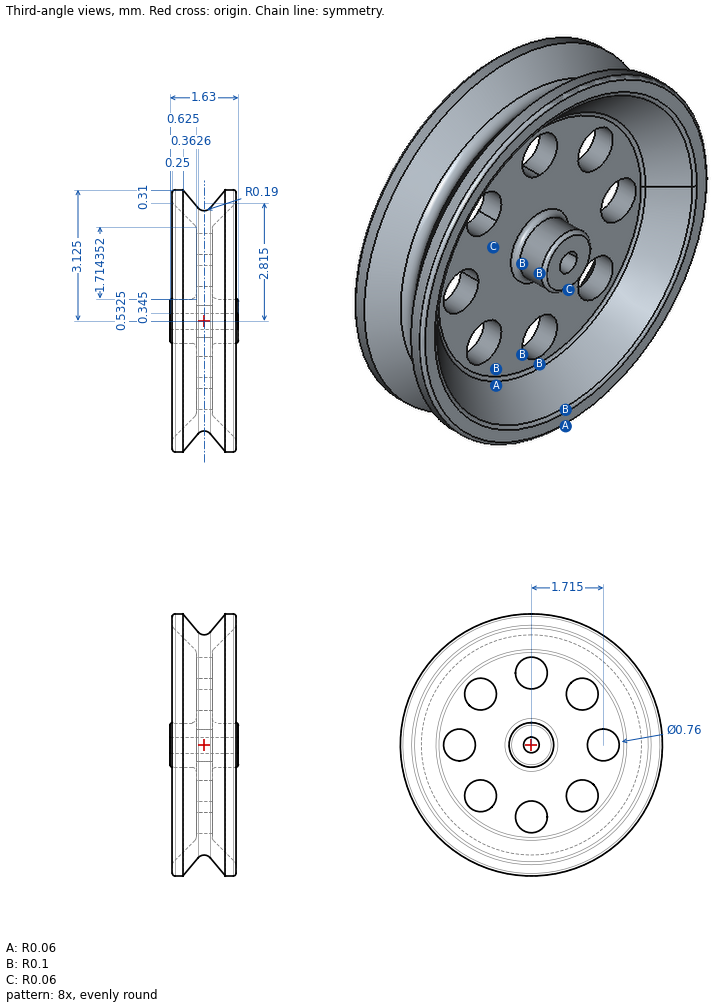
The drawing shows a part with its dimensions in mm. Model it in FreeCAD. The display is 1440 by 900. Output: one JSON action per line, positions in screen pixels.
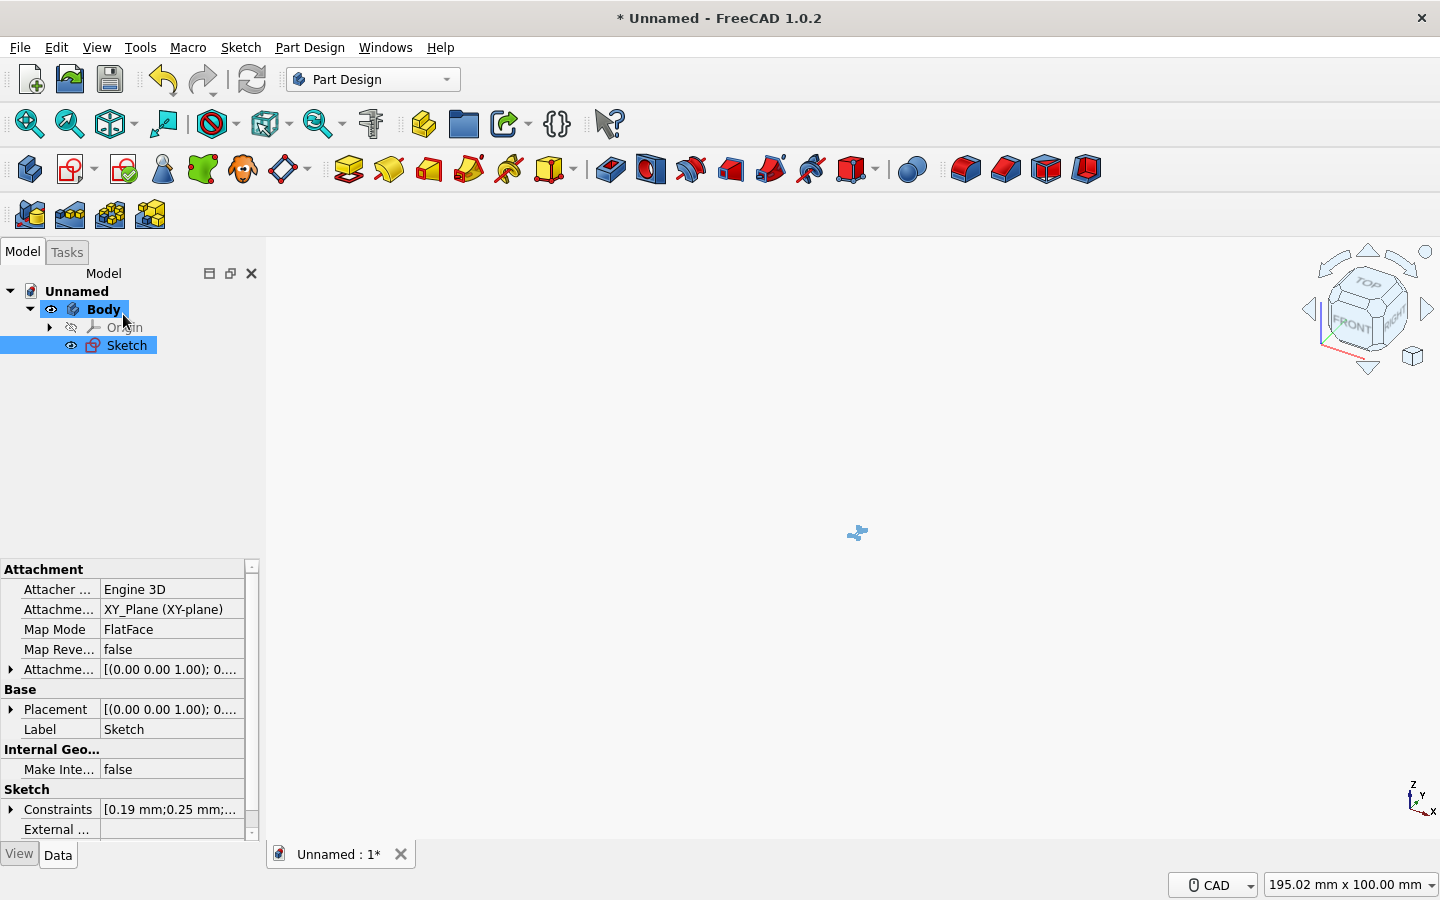
{"action": "left_click", "coordinate": [390, 170]}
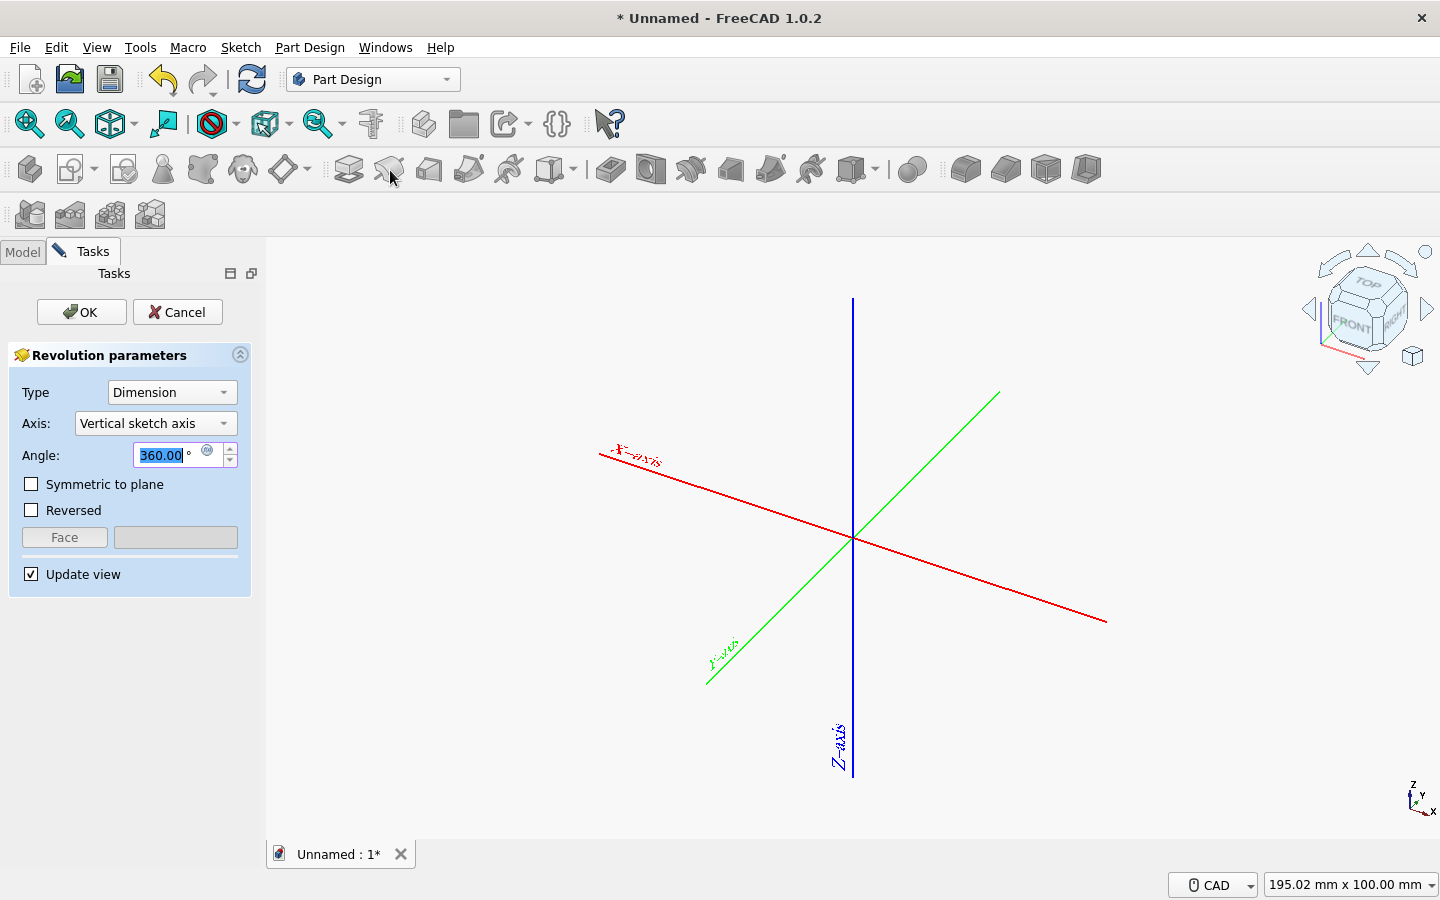
{"action": "left_click", "coordinate": [156, 424]}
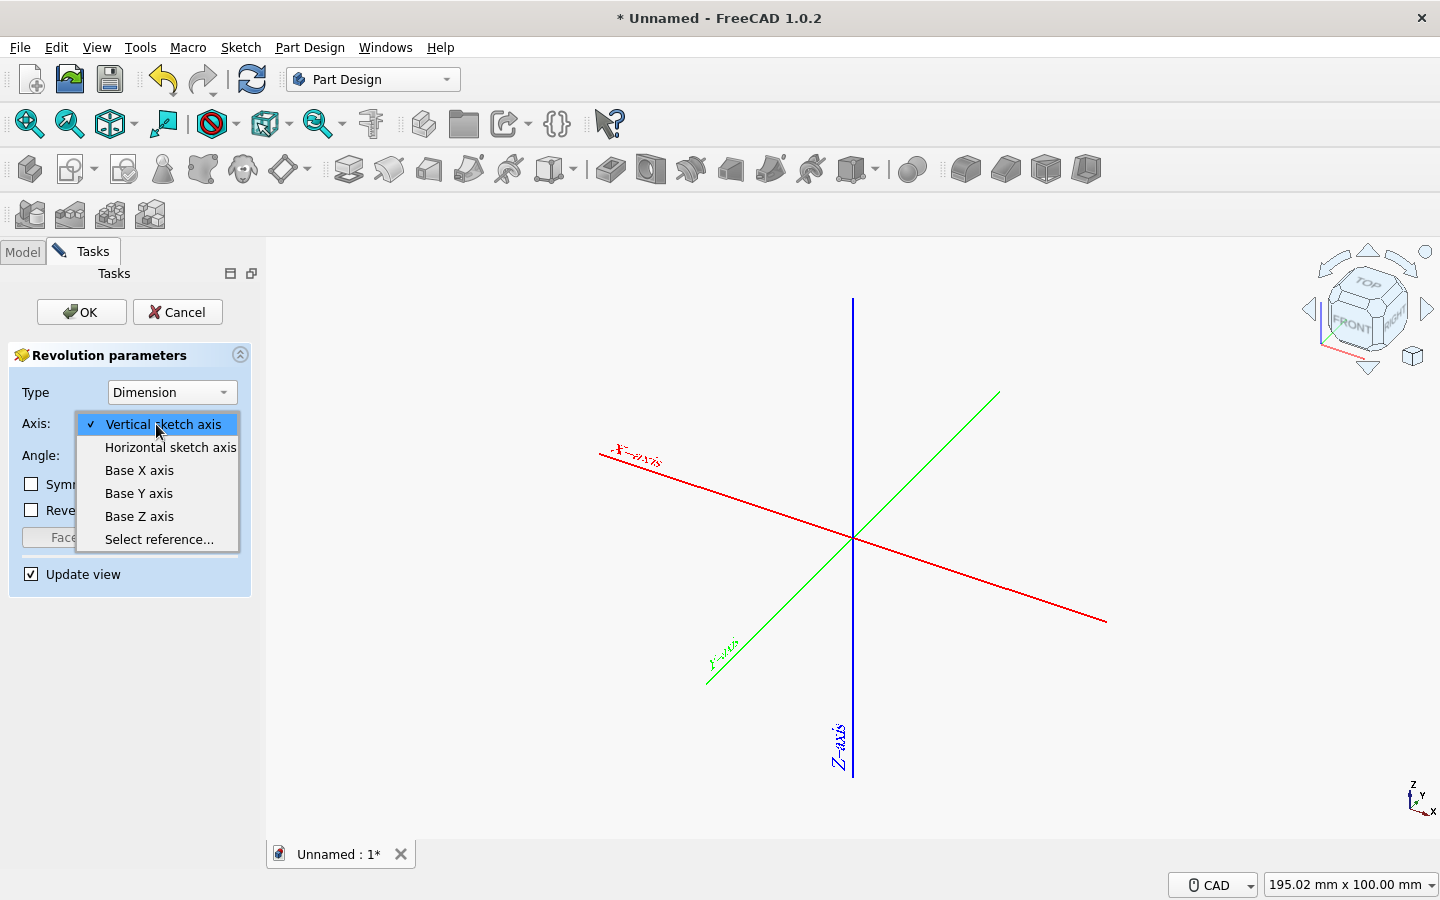
{"action": "left_click", "coordinate": [156, 448]}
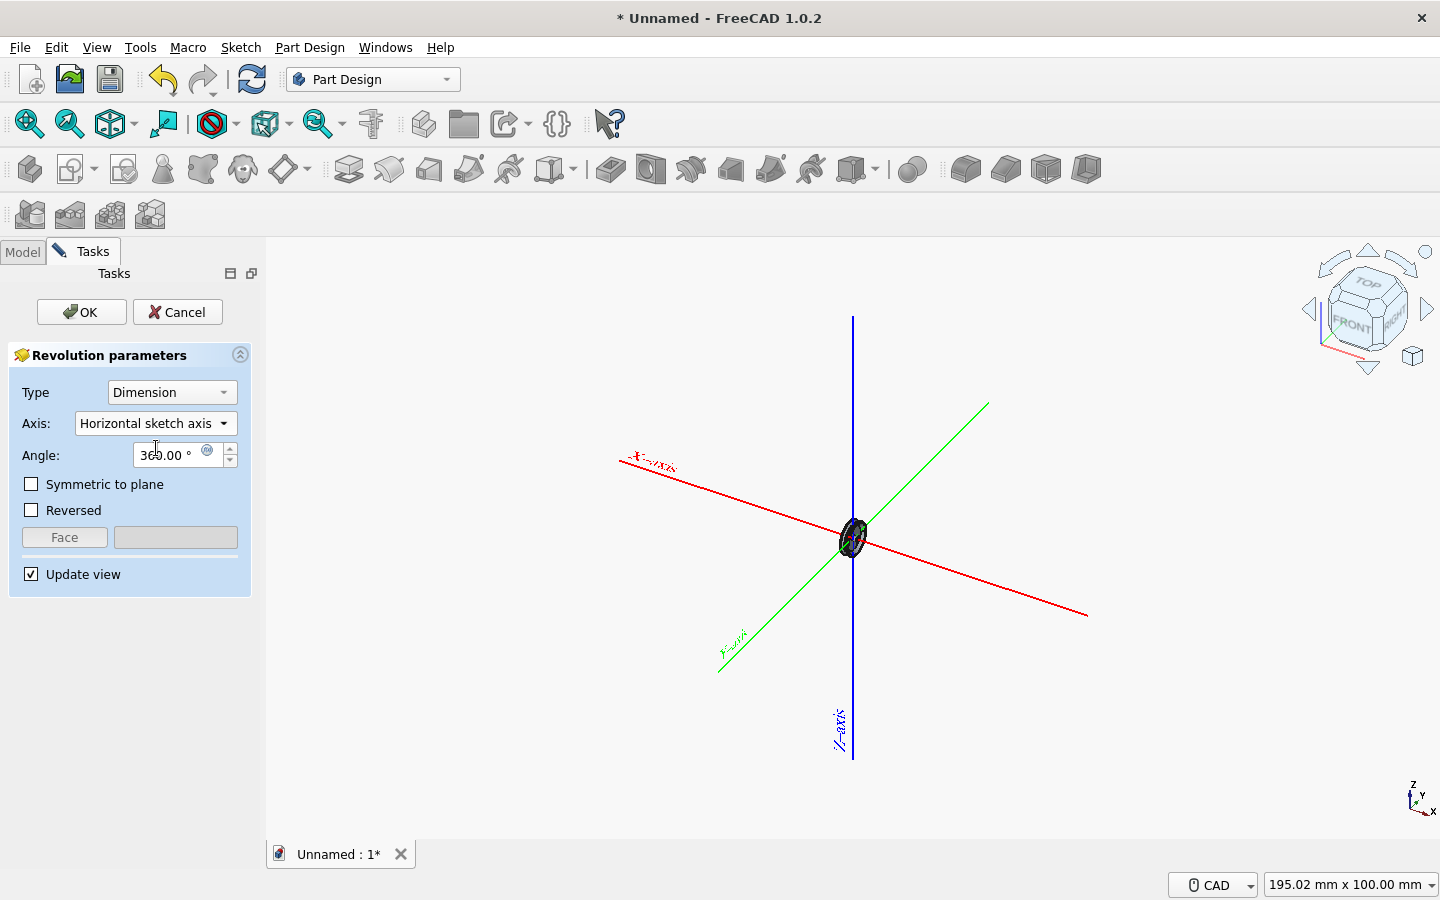
{"action": "left_click", "coordinate": [82, 312]}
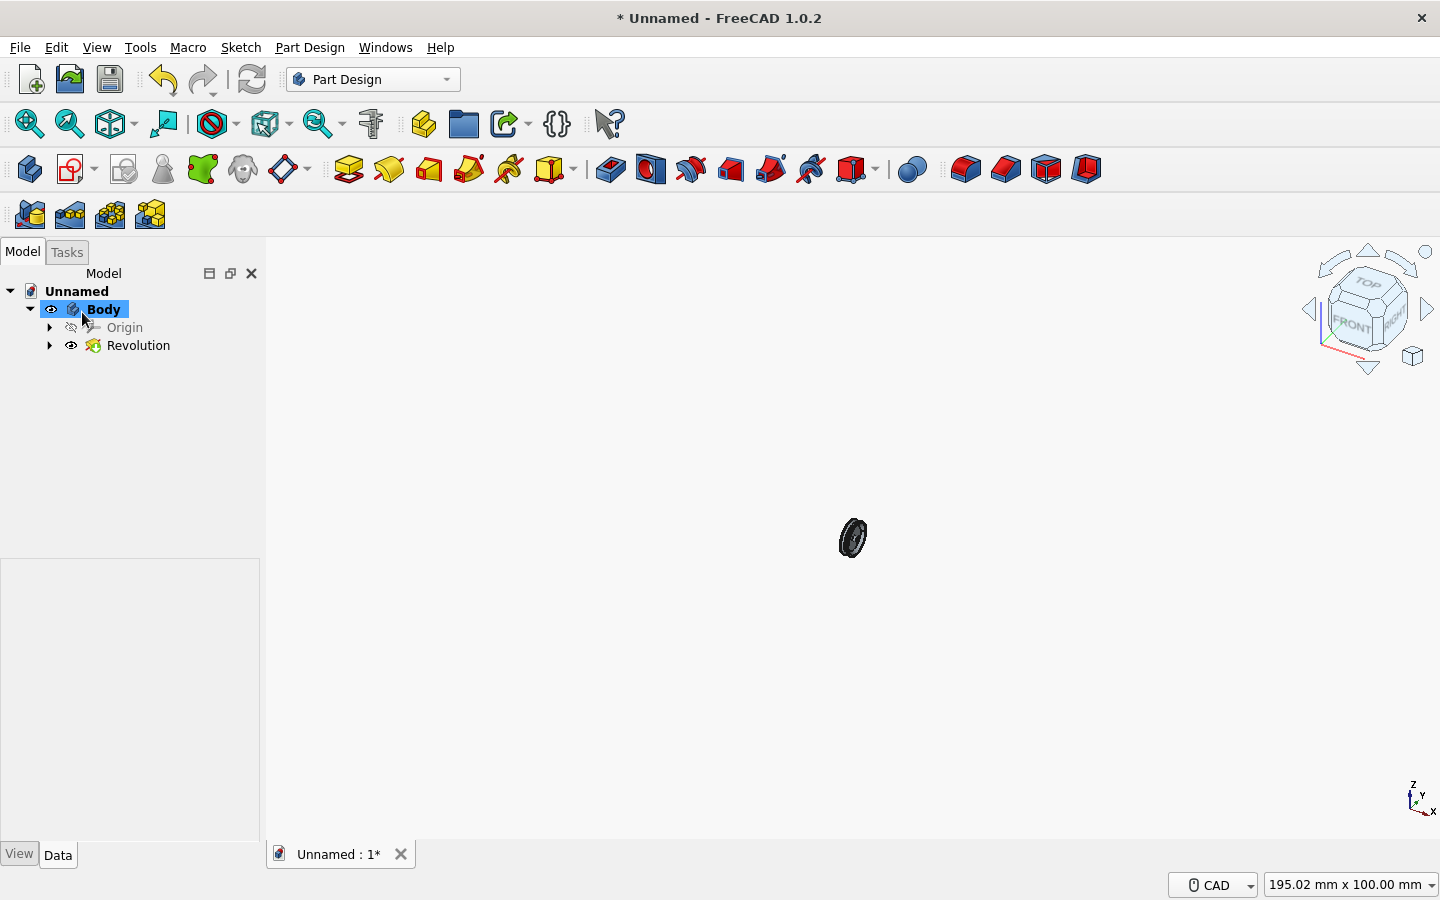
{"action": "left_click", "coordinate": [30, 124]}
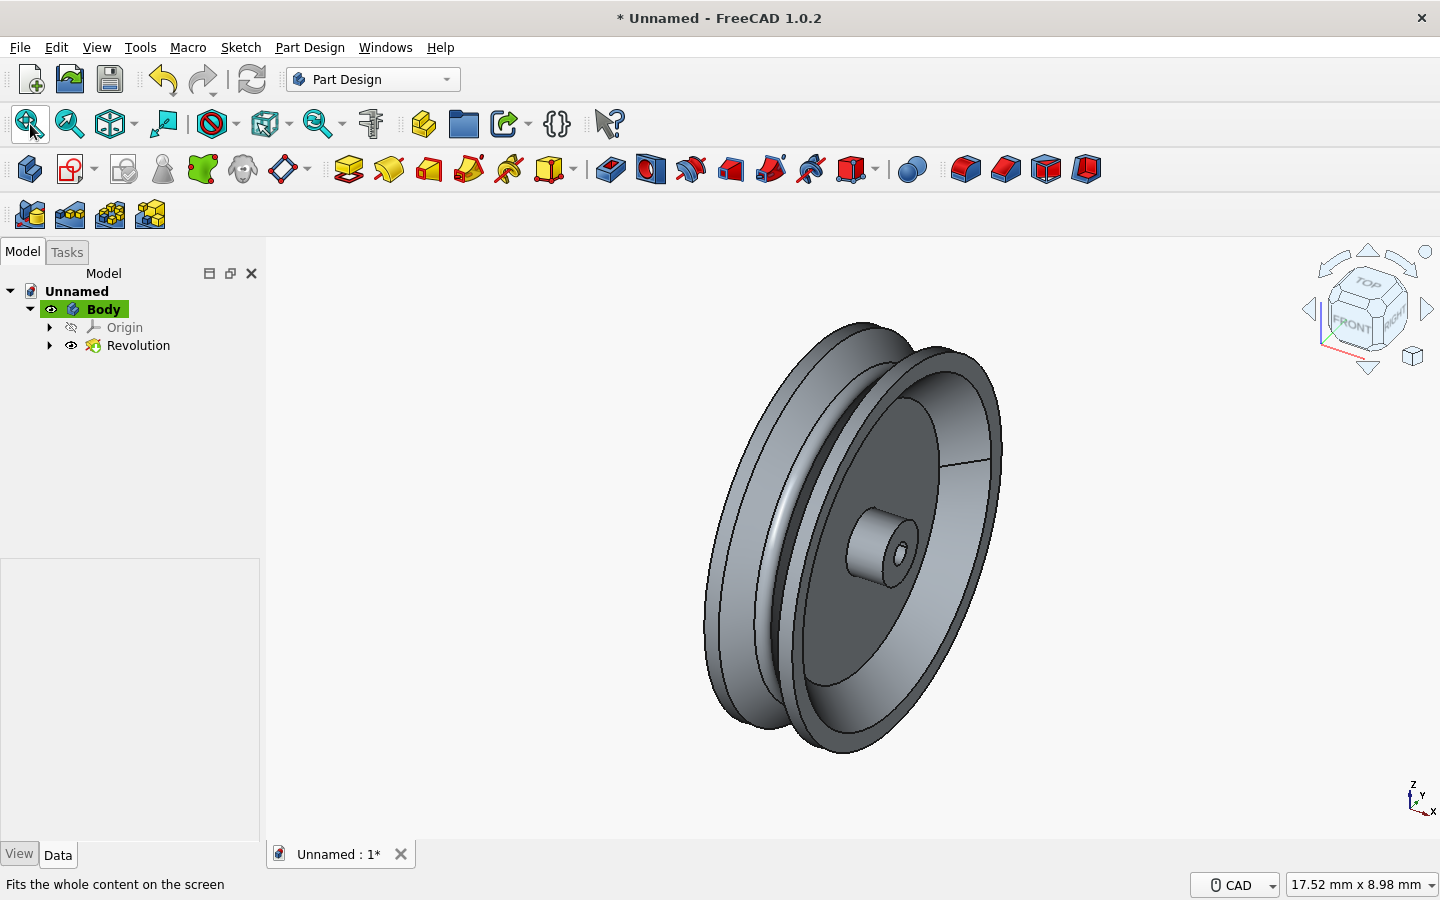
{"action": "left_click", "coordinate": [792, 656]}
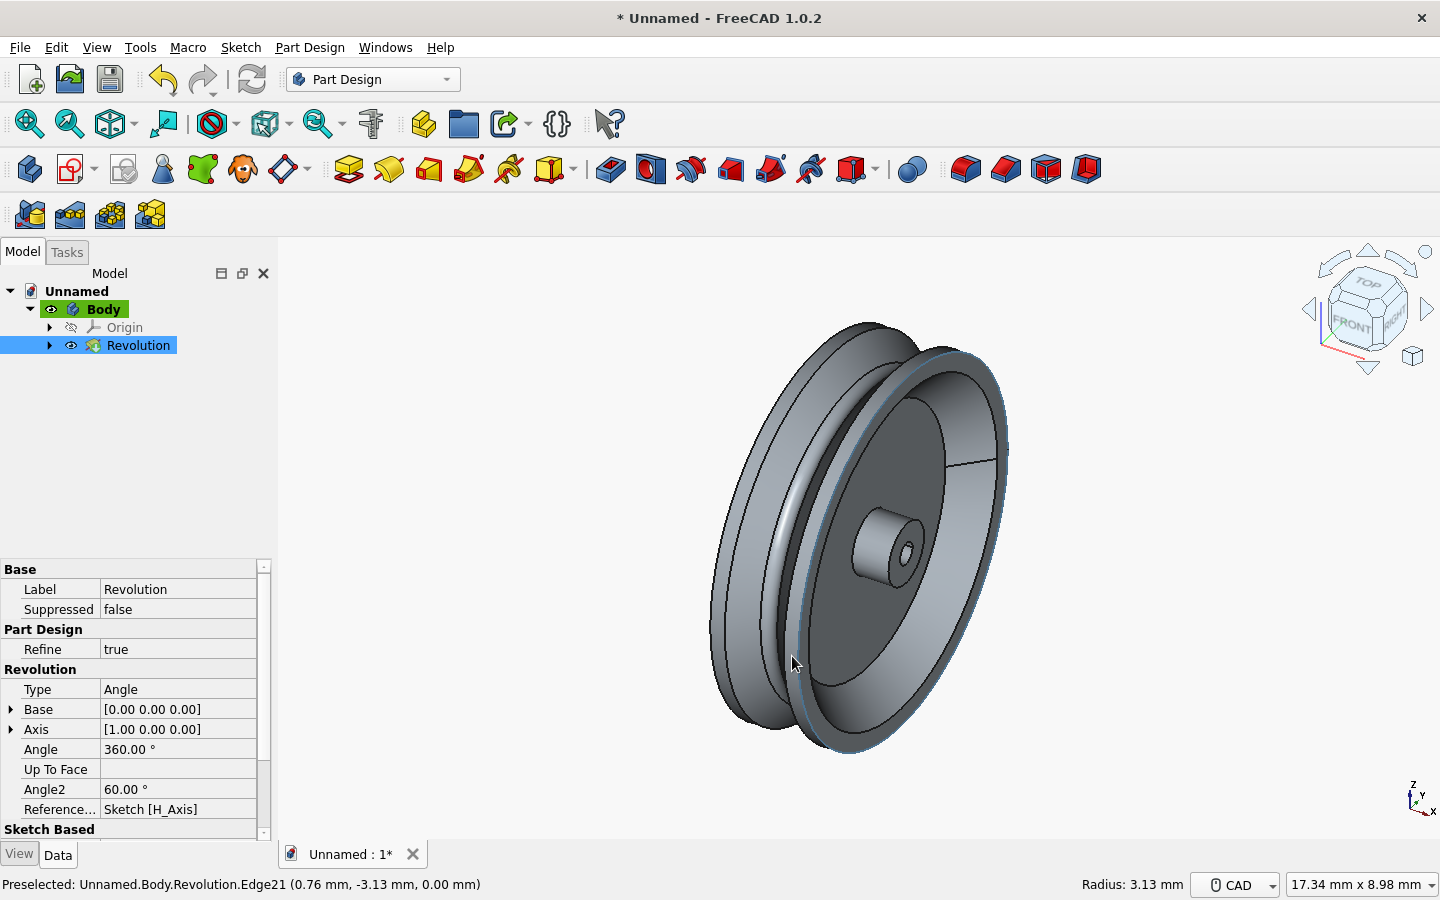
{"action": "key", "text": "0"}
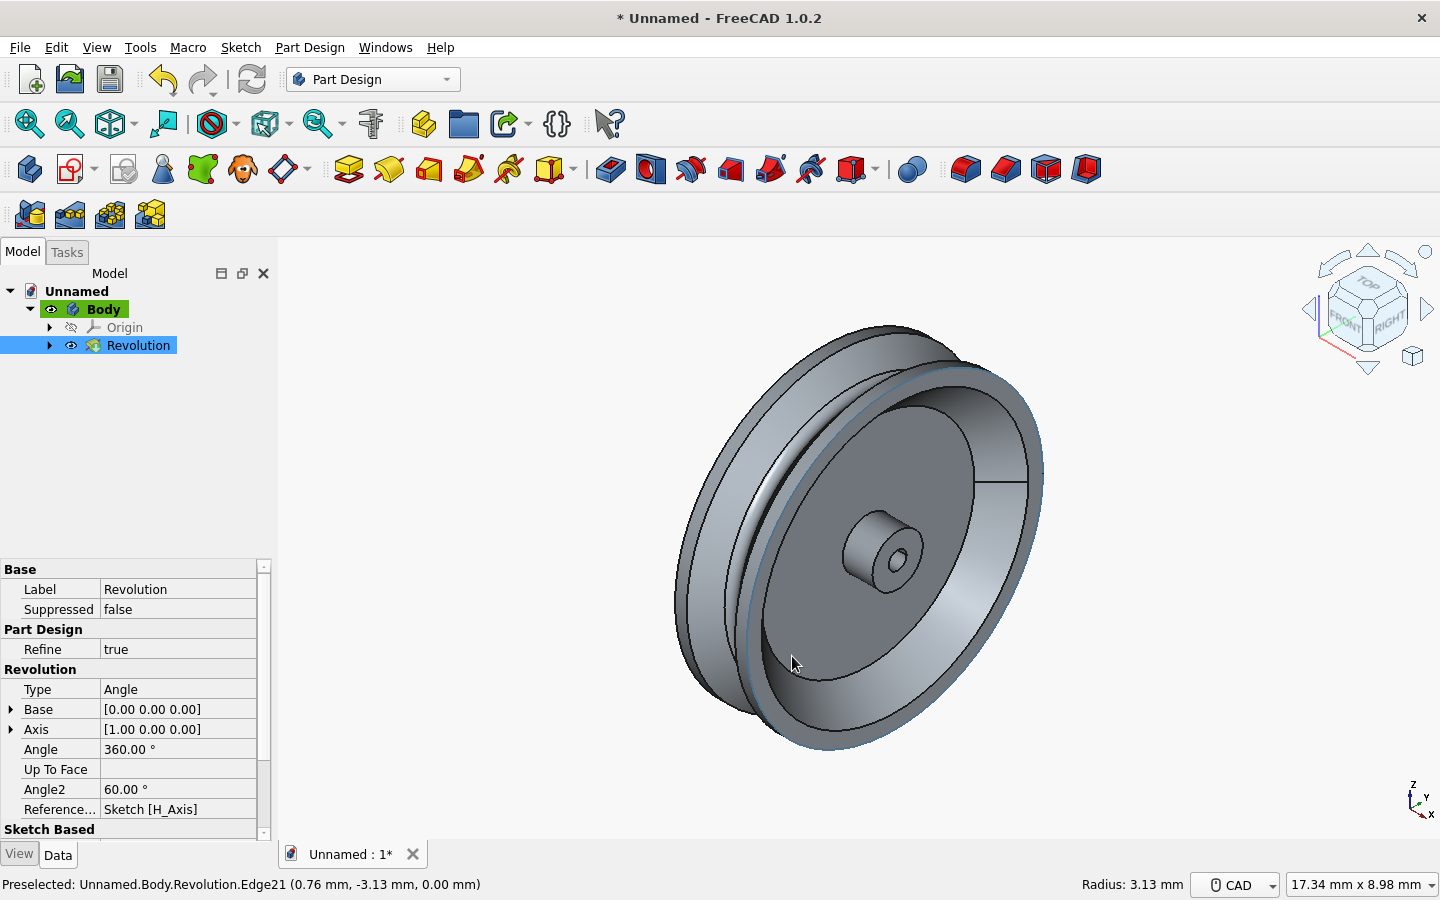
{"action": "key", "text": "2"}